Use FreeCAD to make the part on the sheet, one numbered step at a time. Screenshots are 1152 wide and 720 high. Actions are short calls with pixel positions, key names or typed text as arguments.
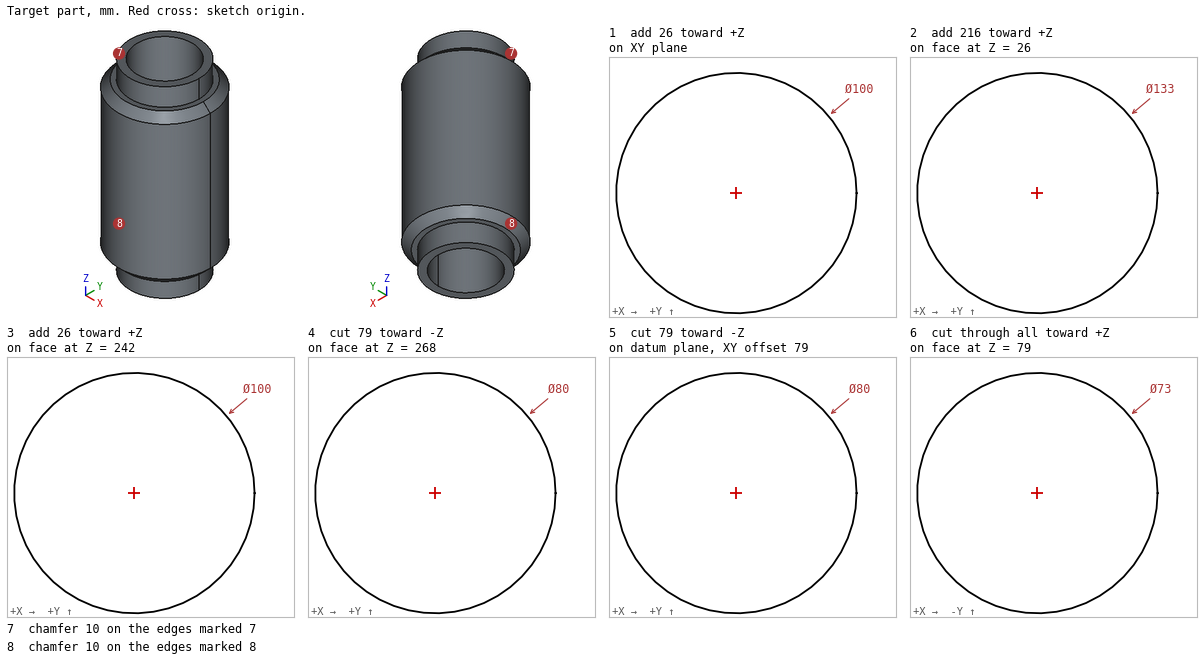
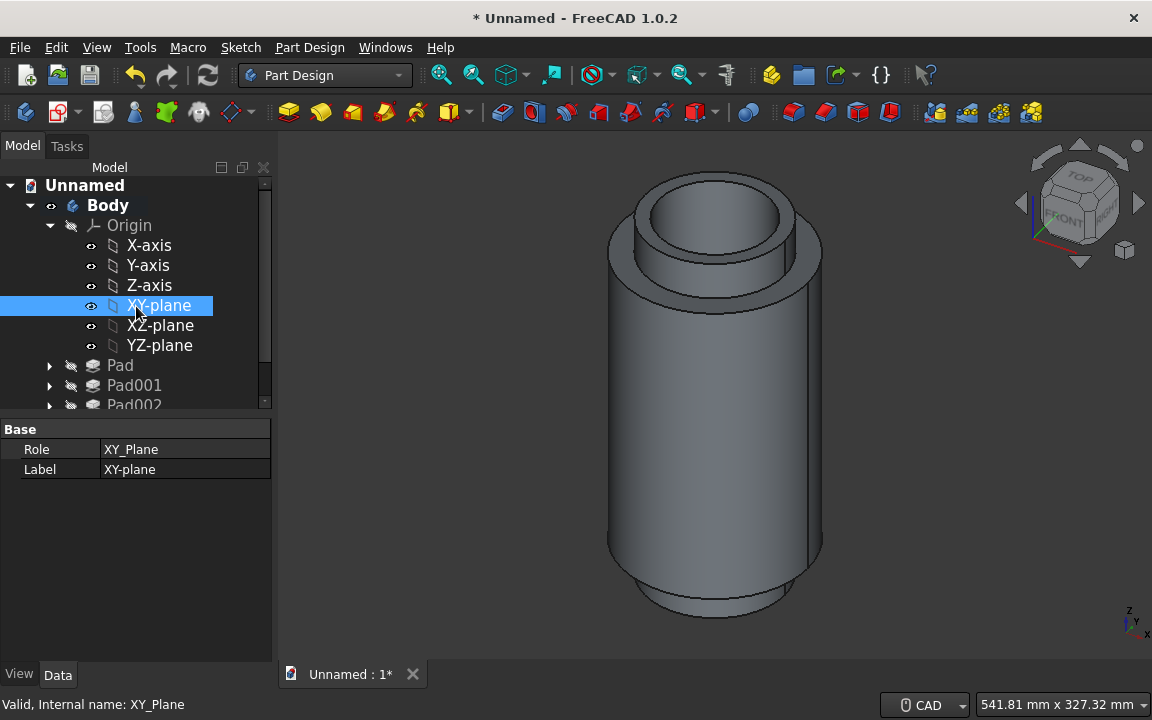
click(232, 112)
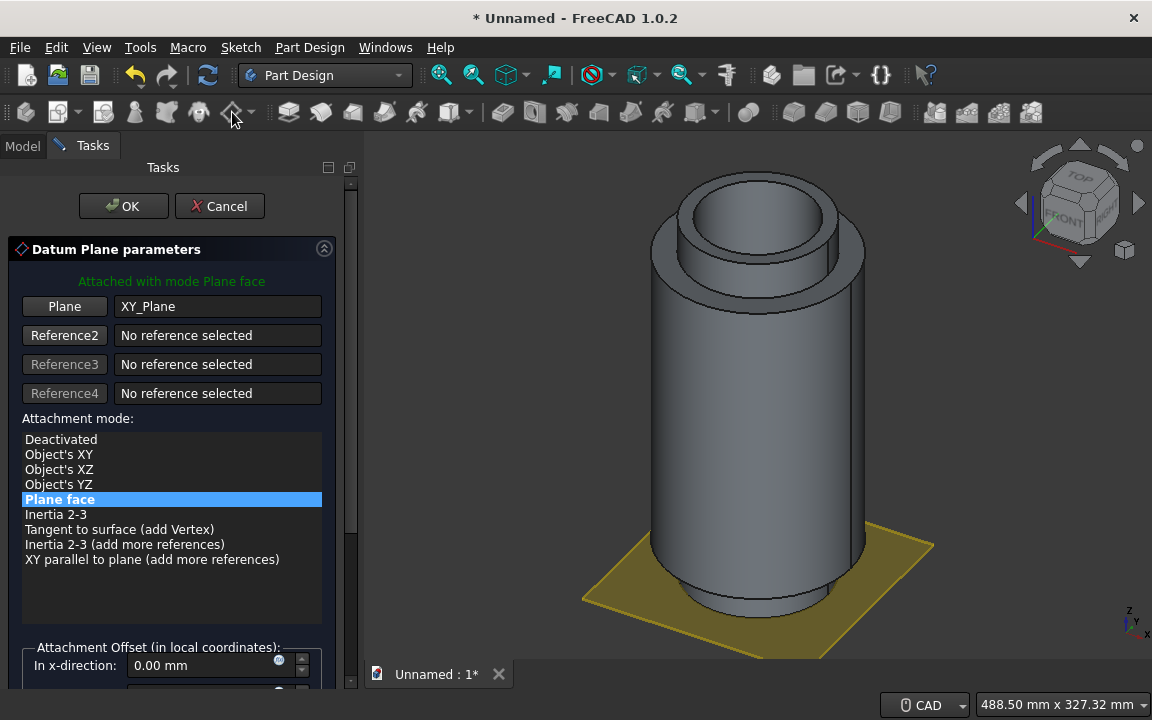
scroll(351, 432, down, 2)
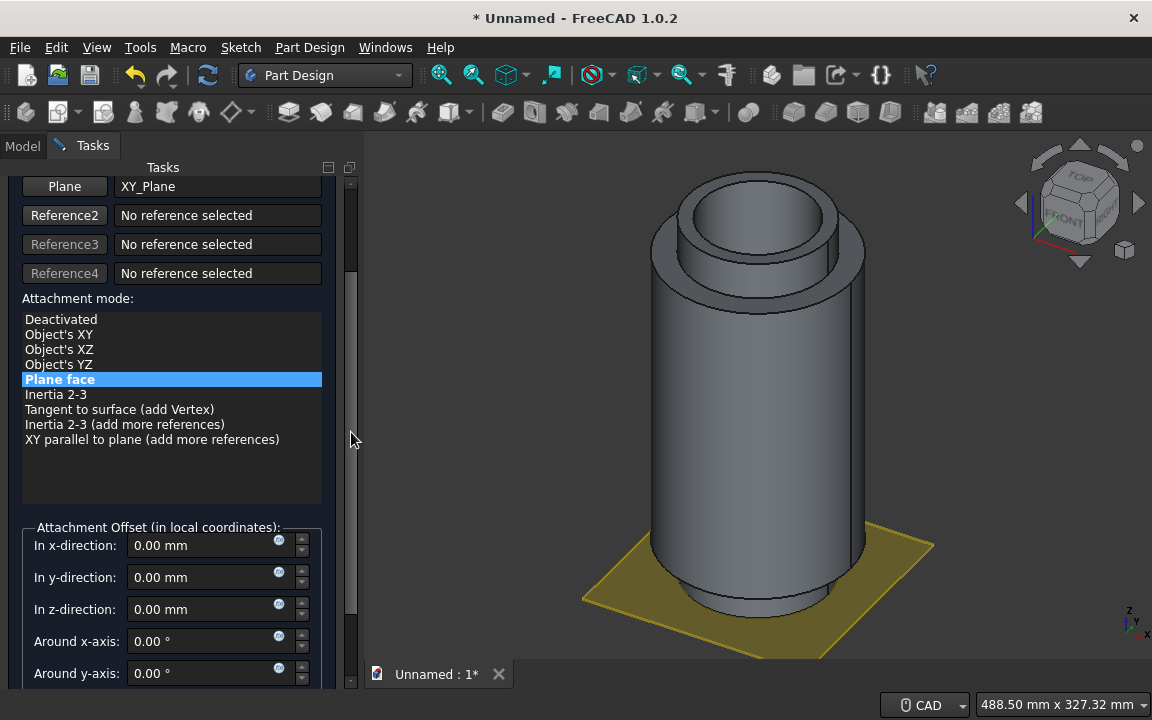
triple_click(210, 609)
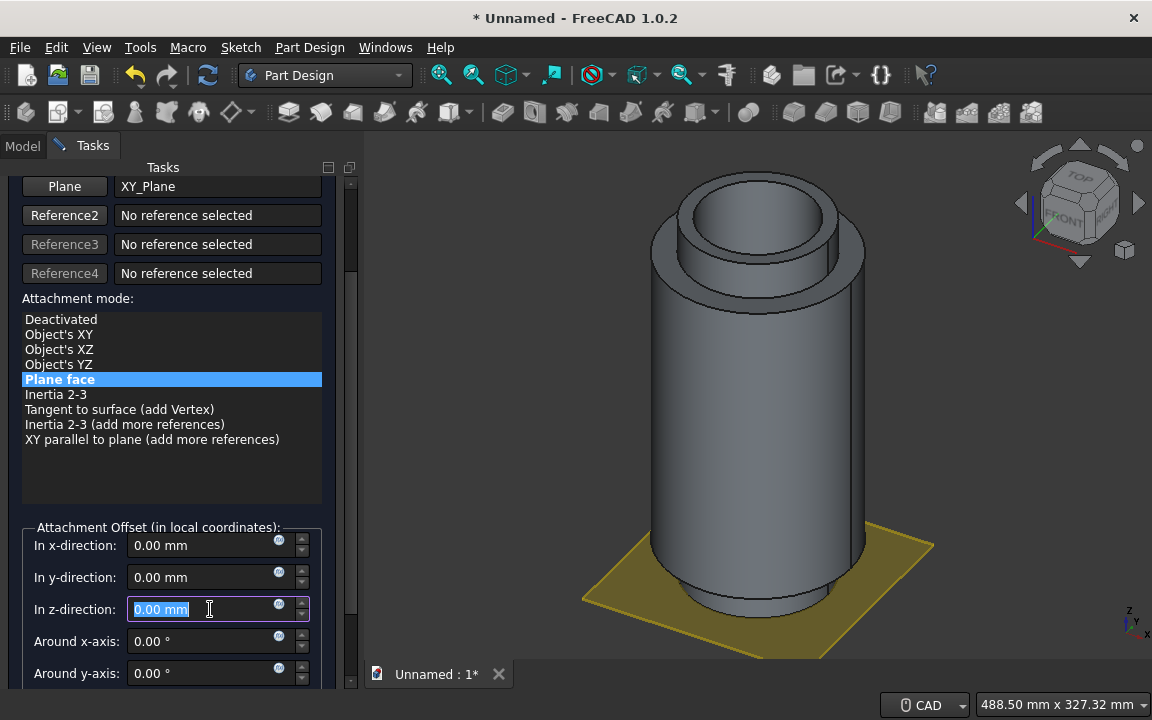
text(79)
key(Tab)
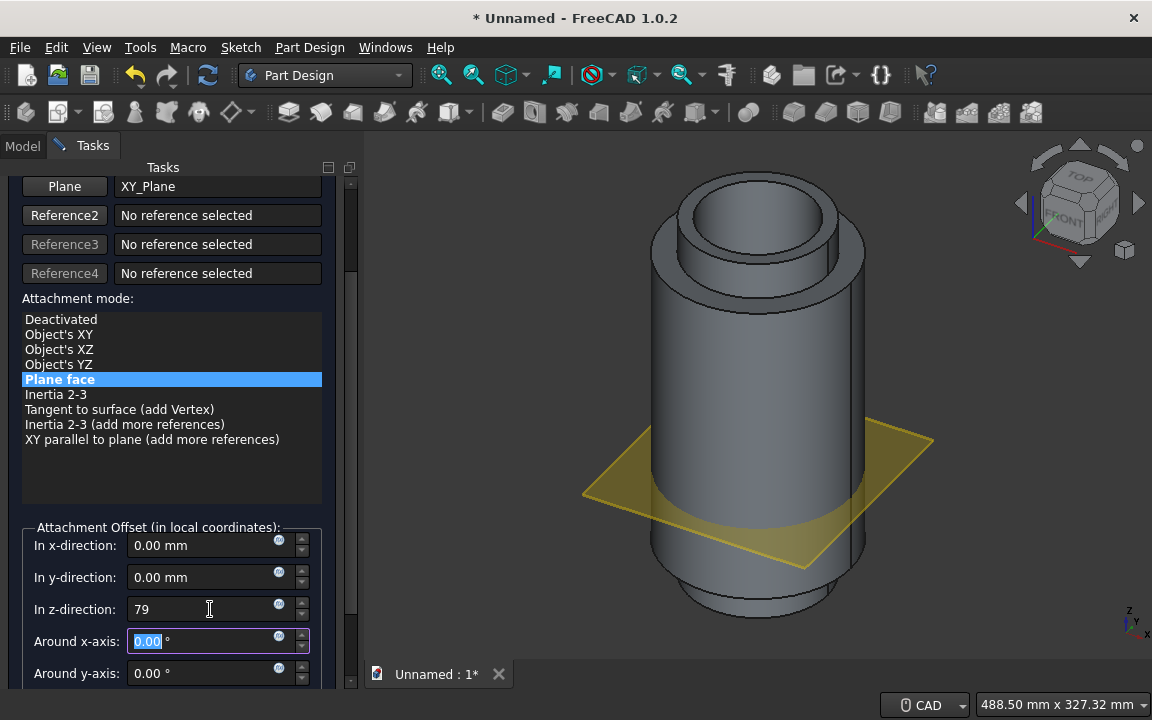
scroll(351, 432, up, 3)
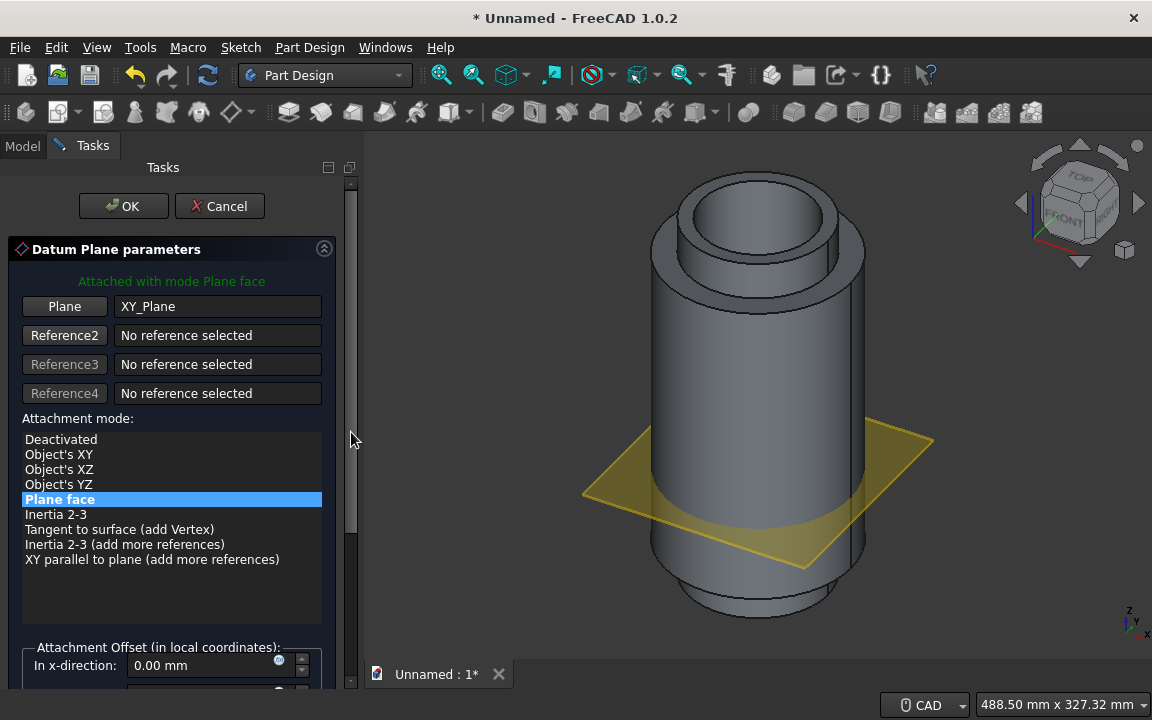
click(124, 206)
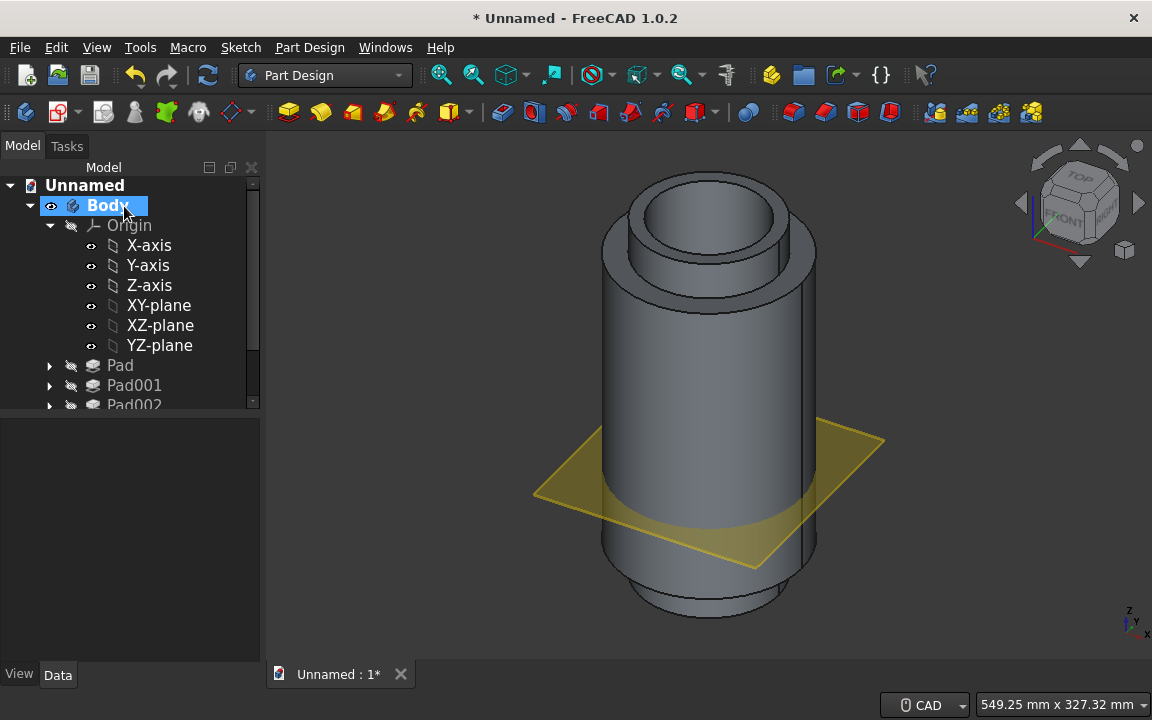
scroll(100, 301, down, 3)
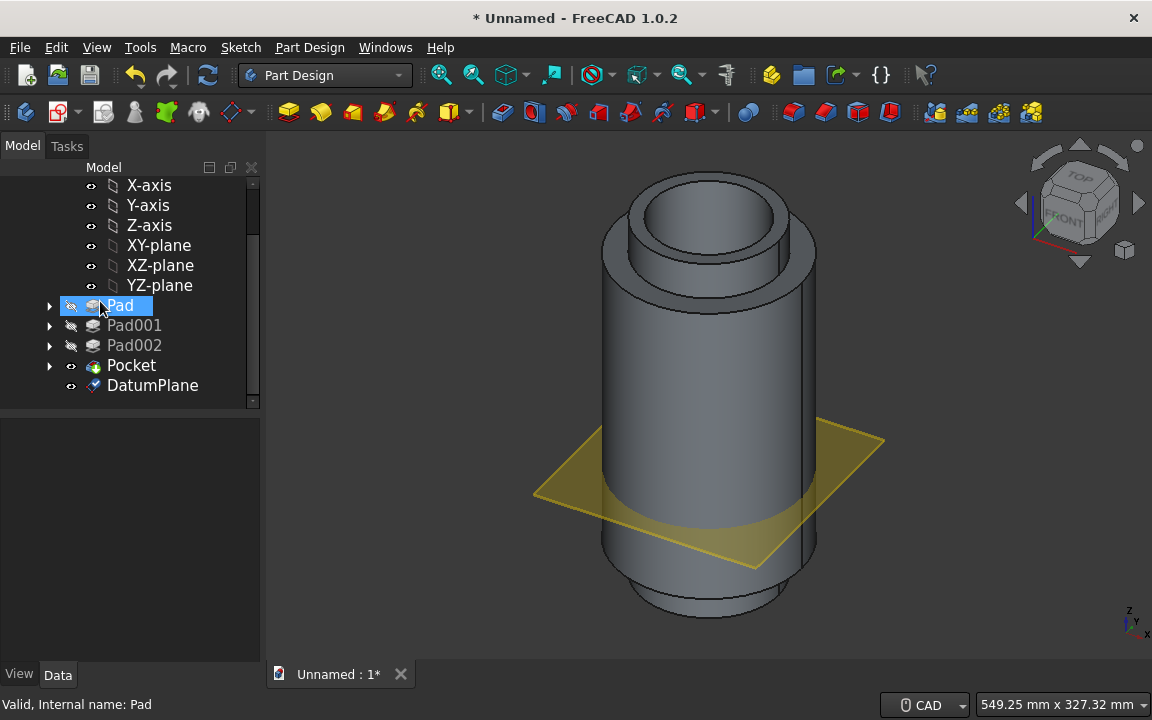
click(116, 386)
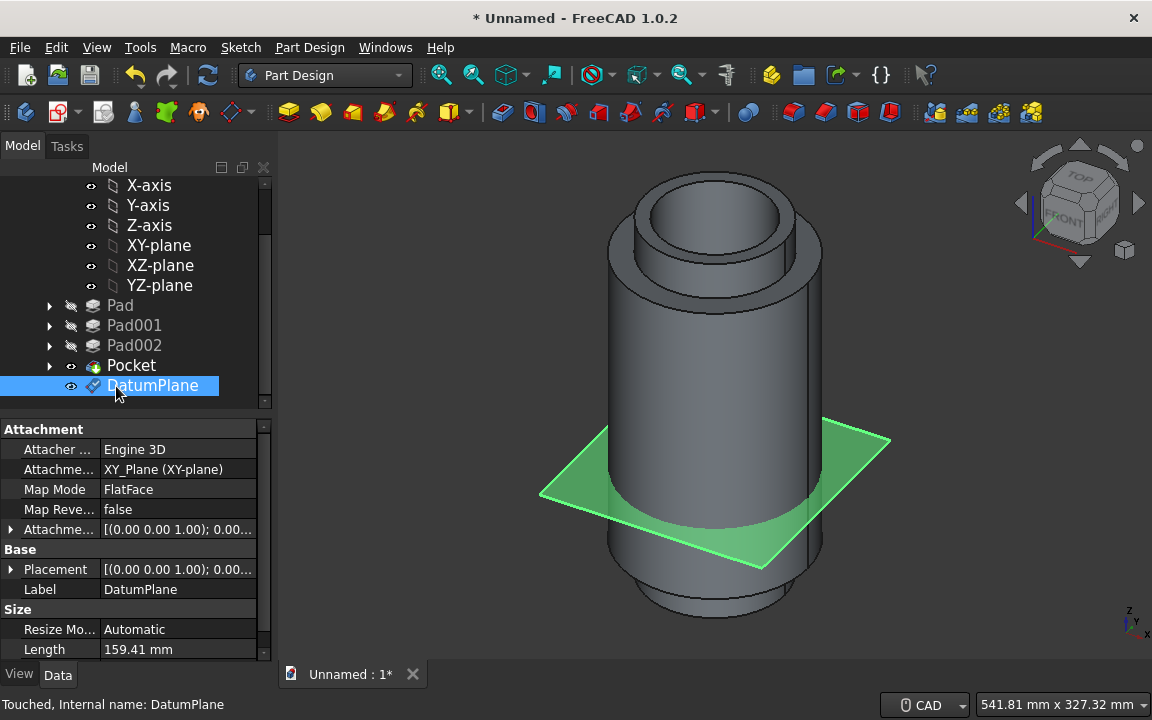
click(58, 112)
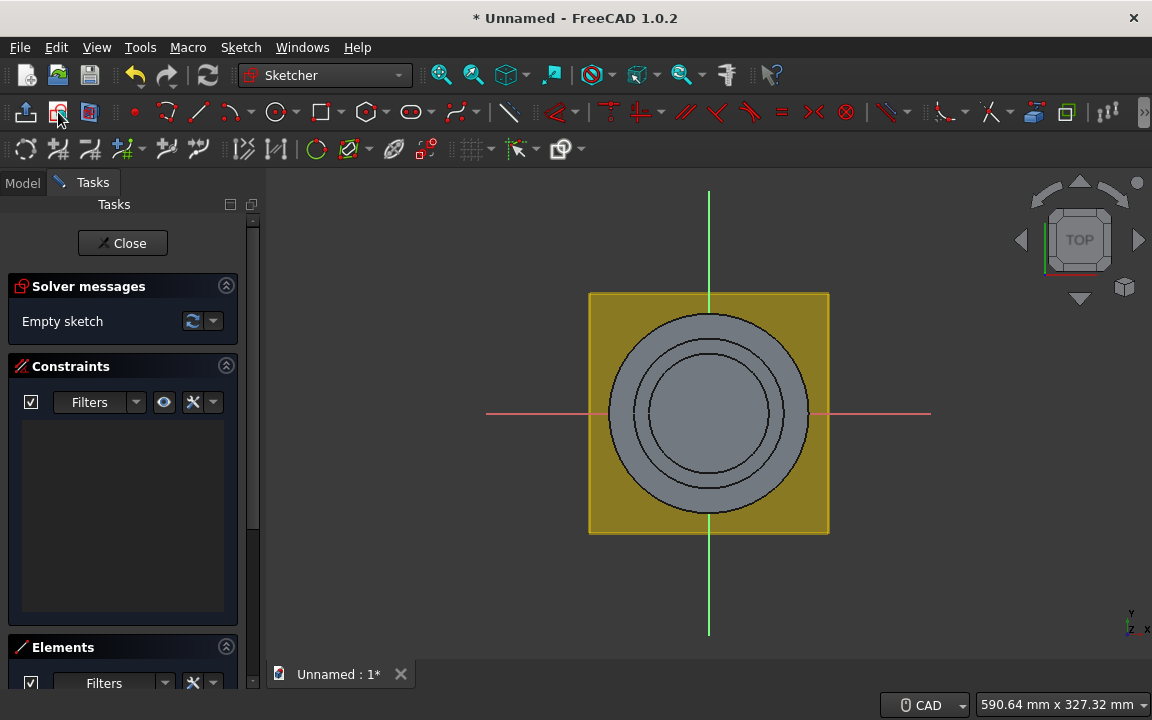
click(90, 112)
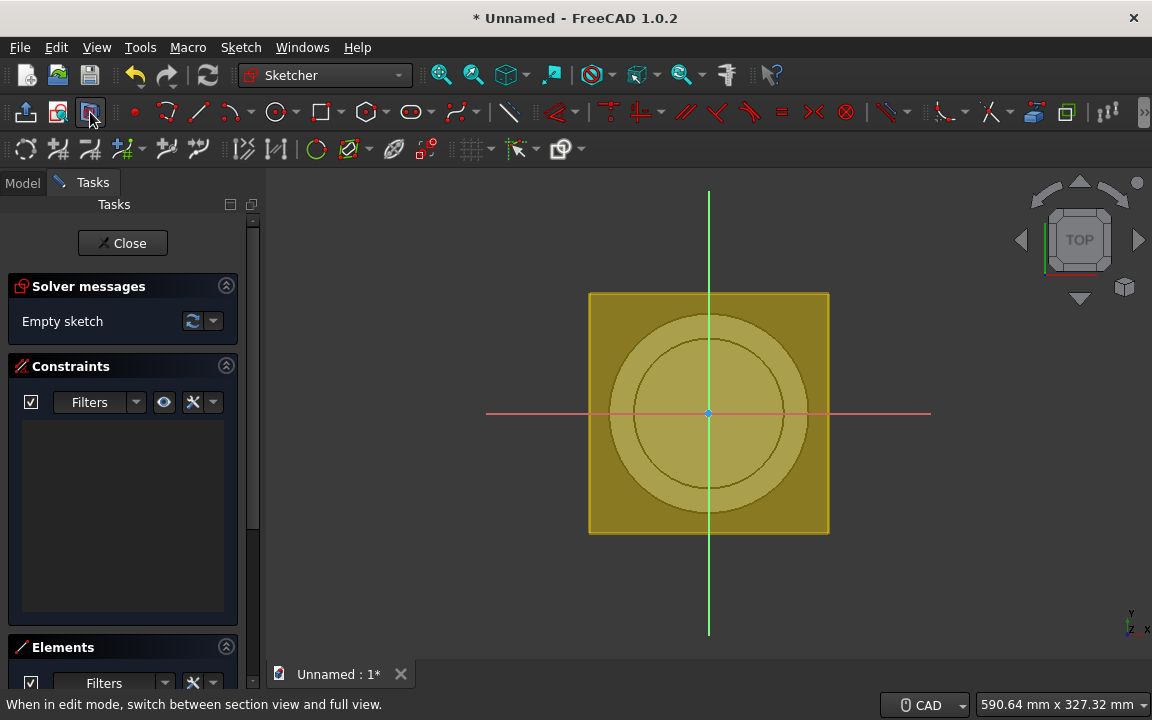
scroll(749, 414, up, 5)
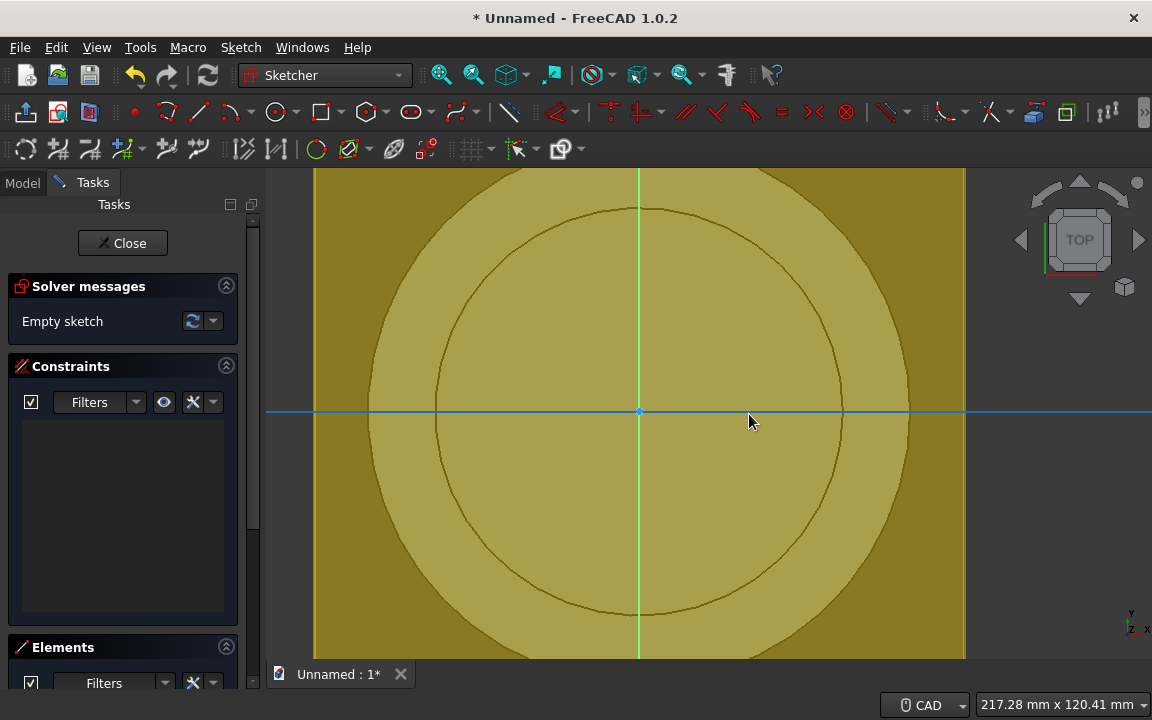
key(g)
key(c)